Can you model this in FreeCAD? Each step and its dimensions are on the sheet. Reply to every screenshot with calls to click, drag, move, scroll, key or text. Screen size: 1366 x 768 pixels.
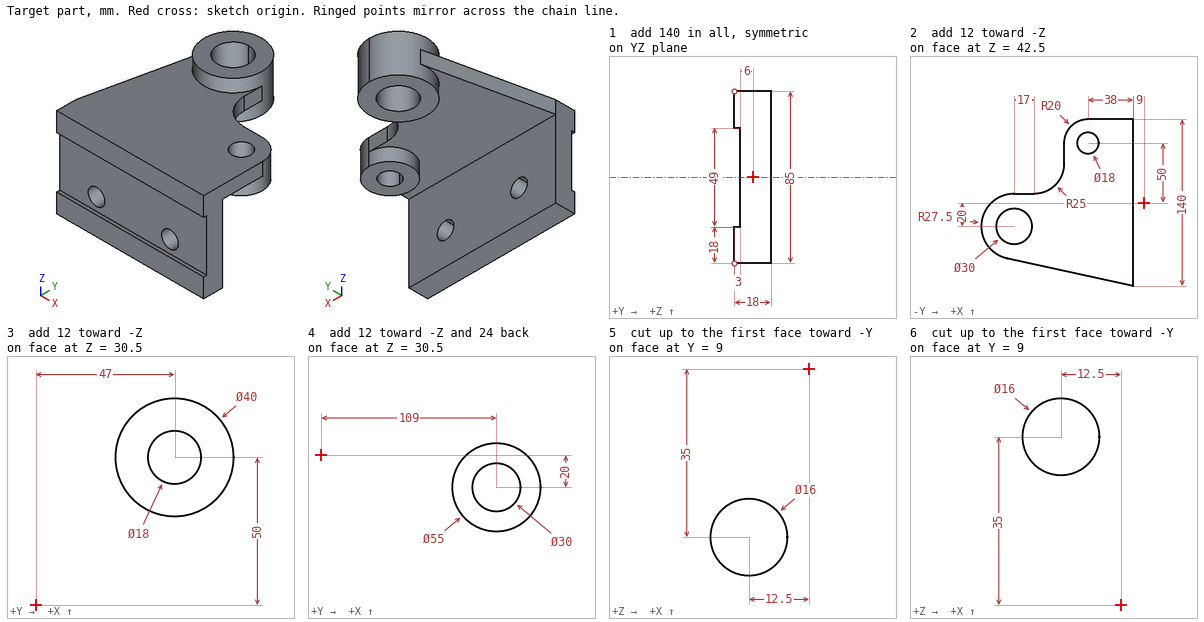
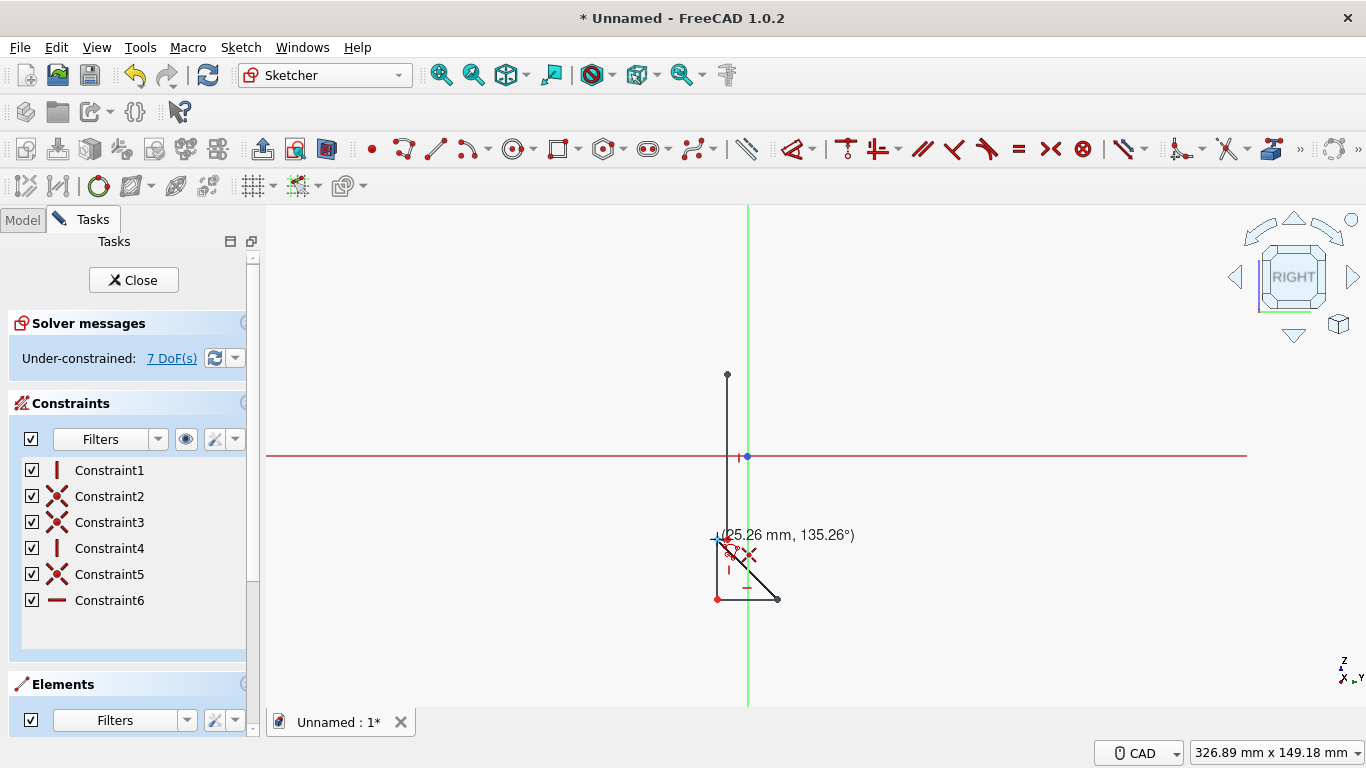
click(778, 313)
click(717, 313)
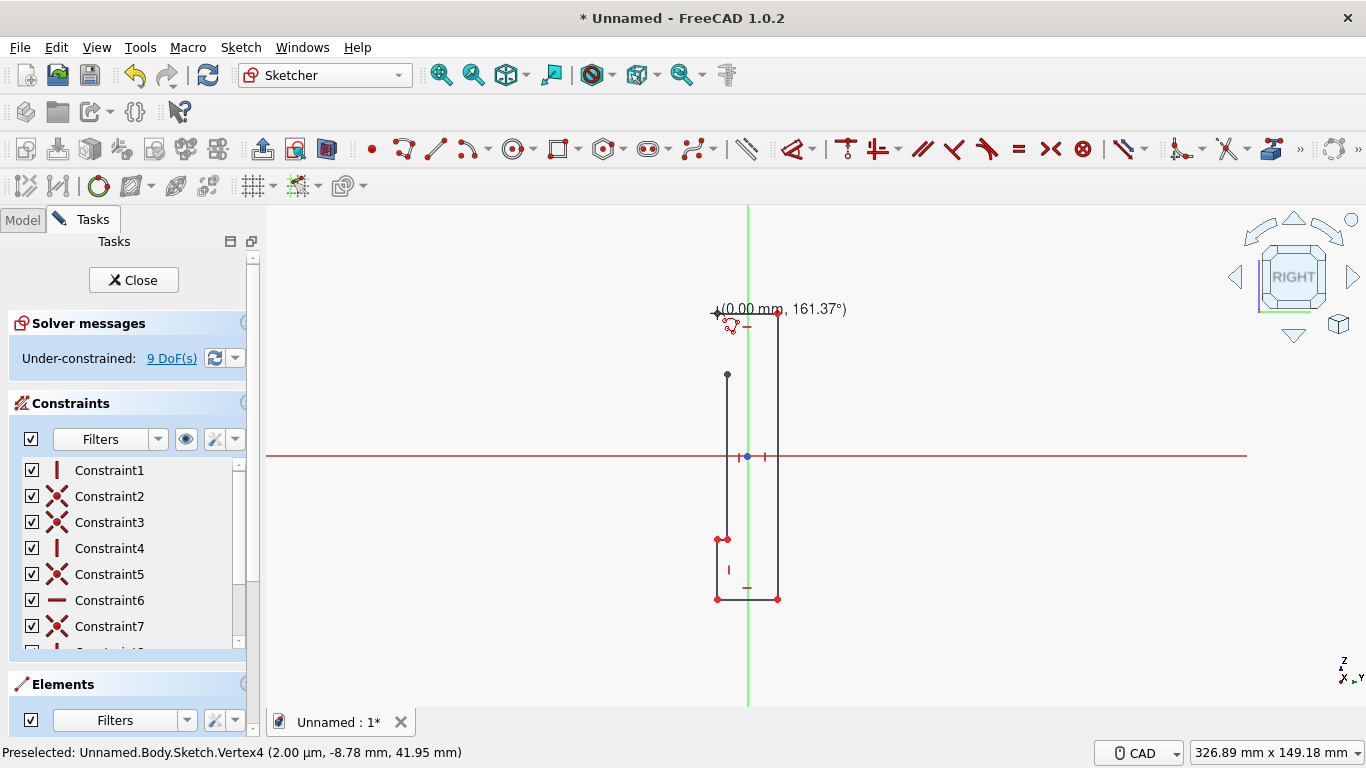
scroll(717, 374, up, 3)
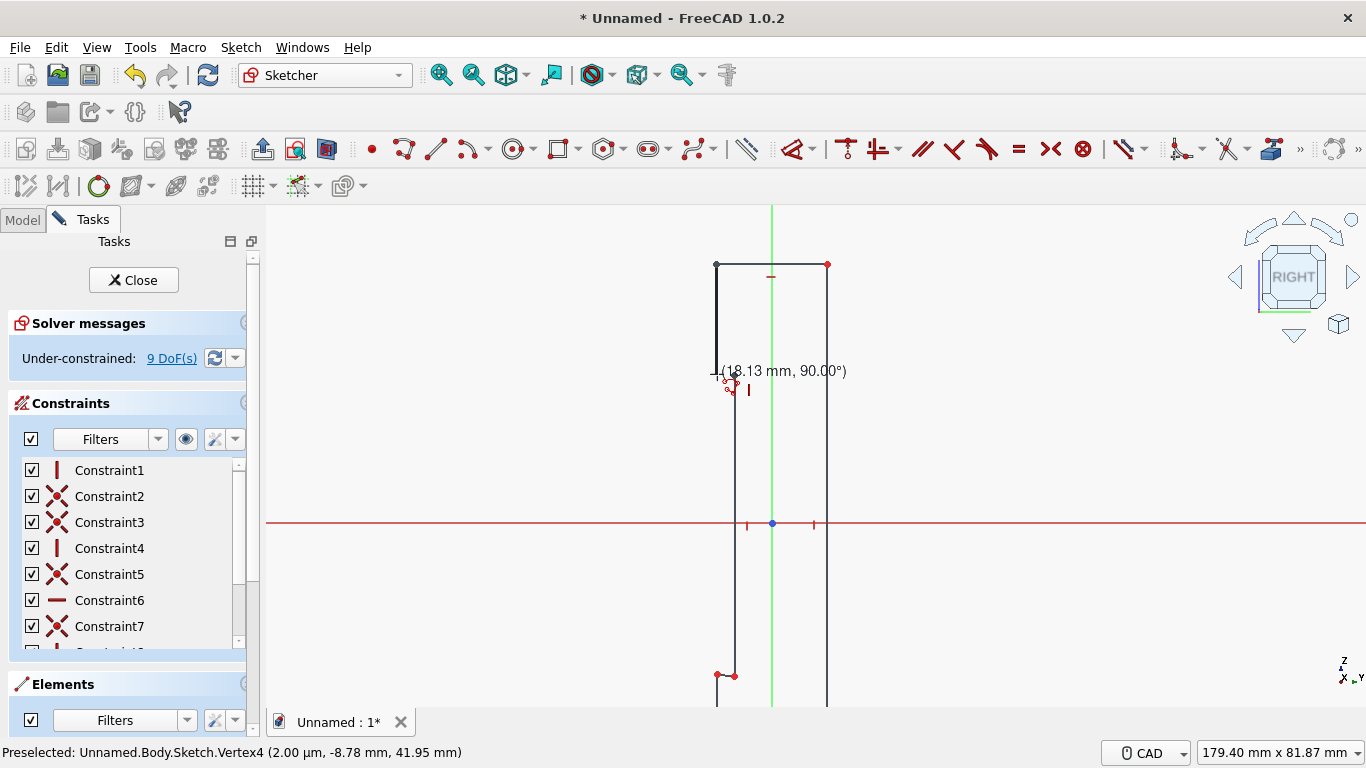
click(717, 373)
click(735, 376)
key(Escape)
key(Escape)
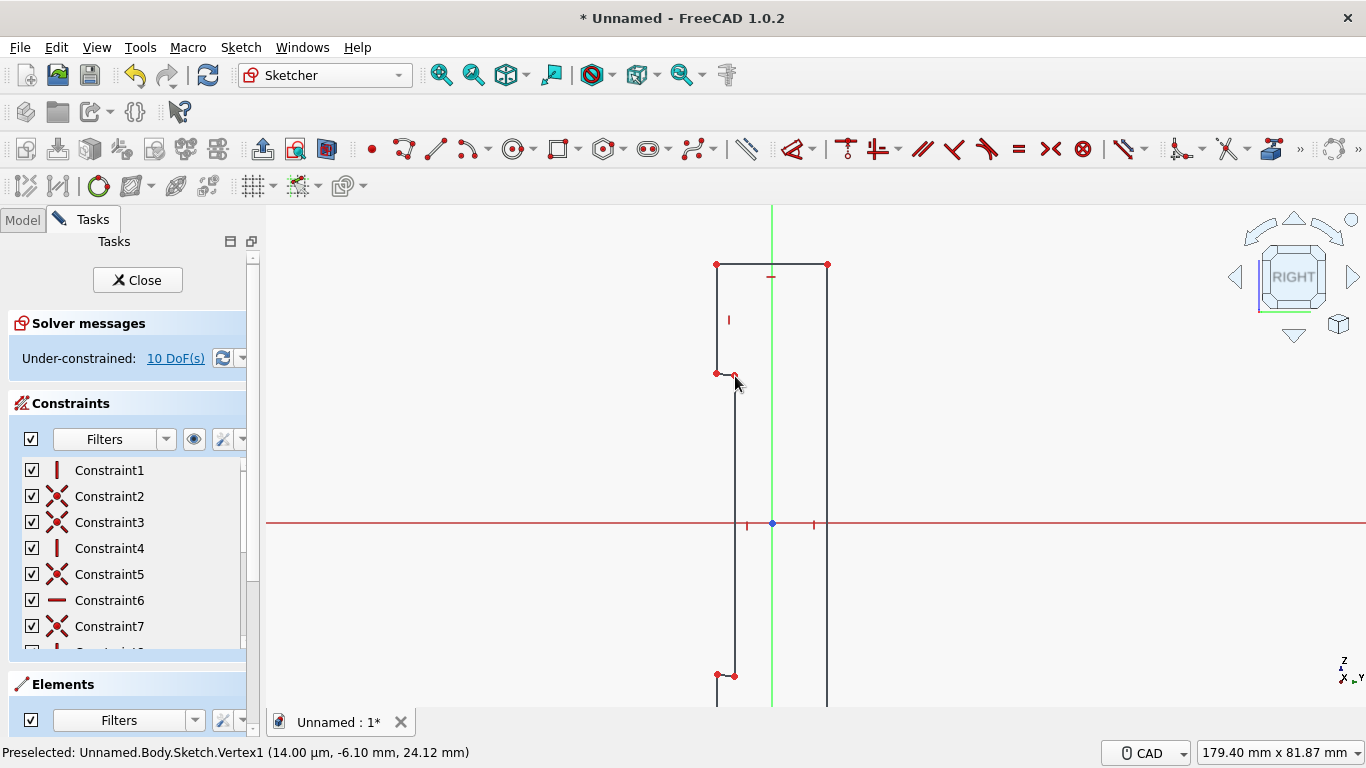
scroll(726, 676, up, 3)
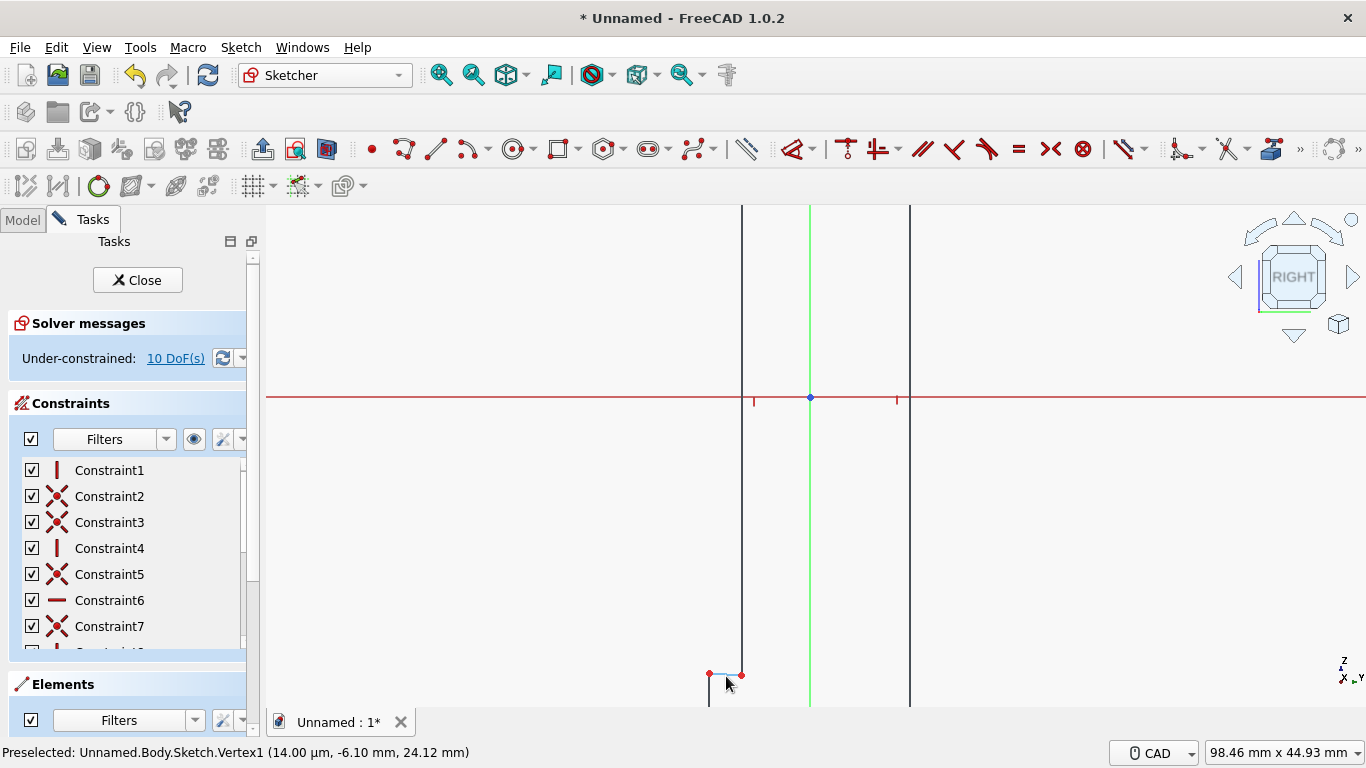
click(726, 674)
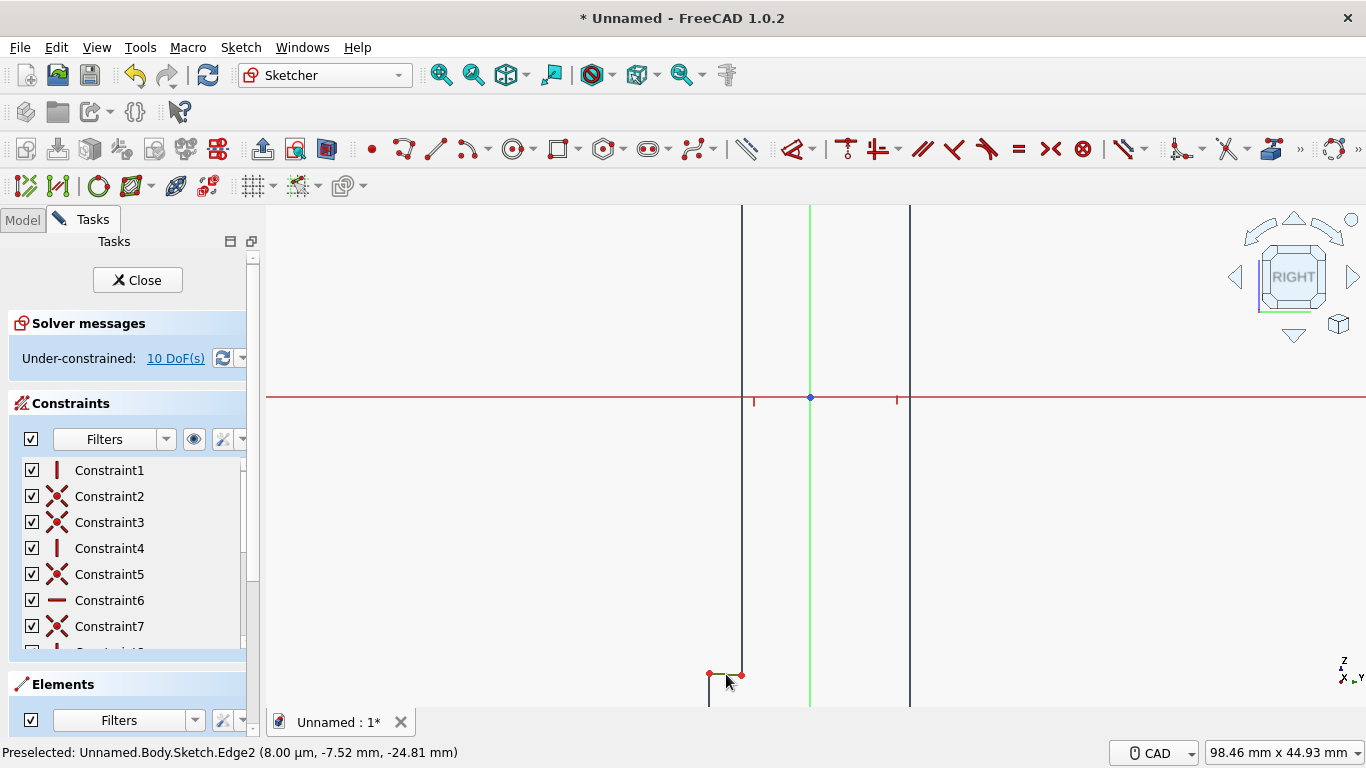
key(h)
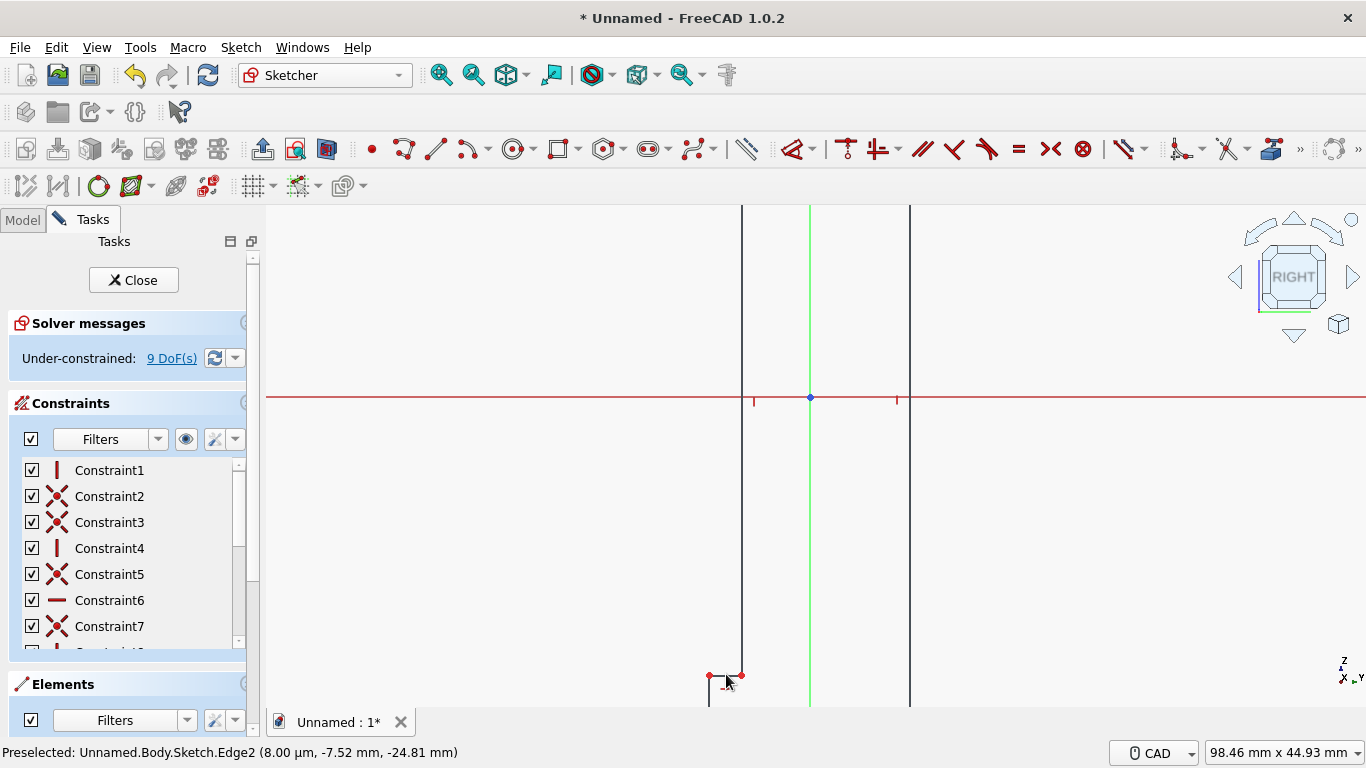
scroll(721, 481, down, 6)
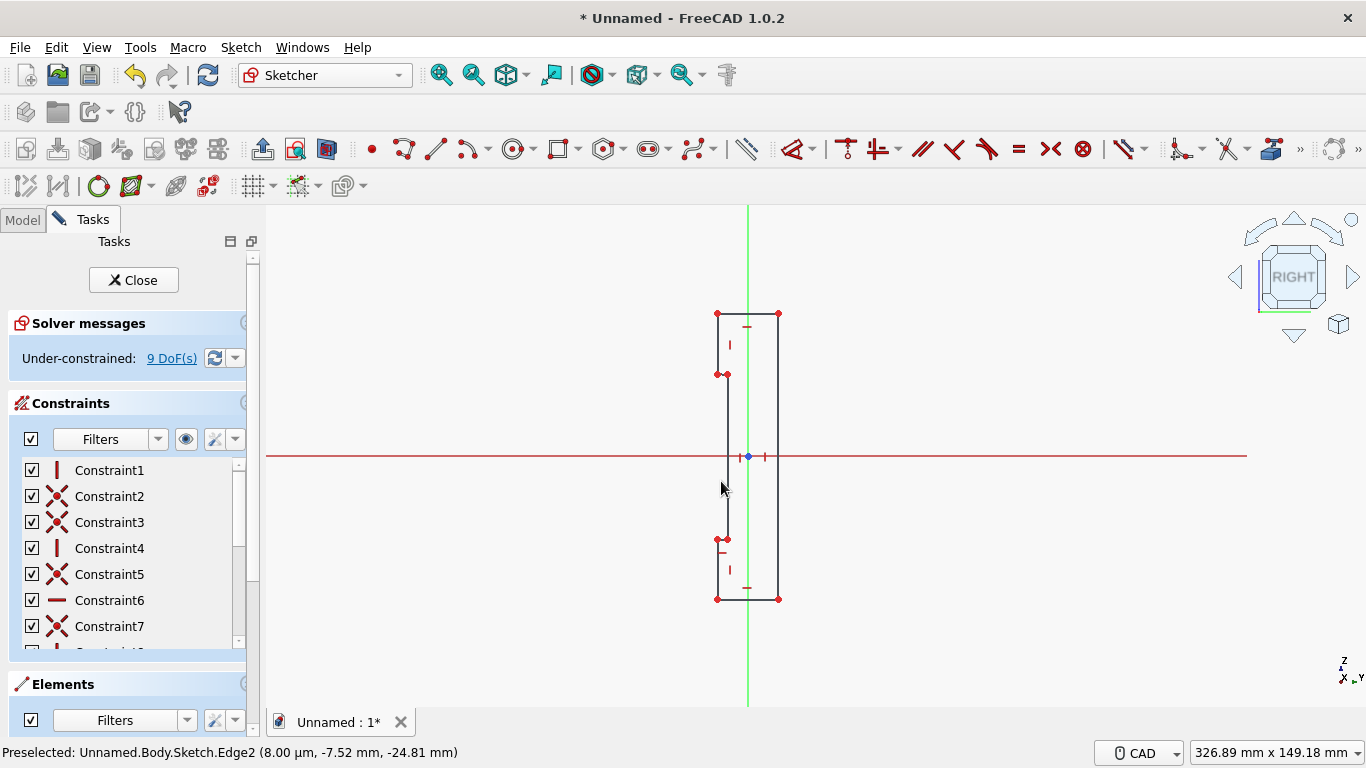
scroll(721, 374, up, 8)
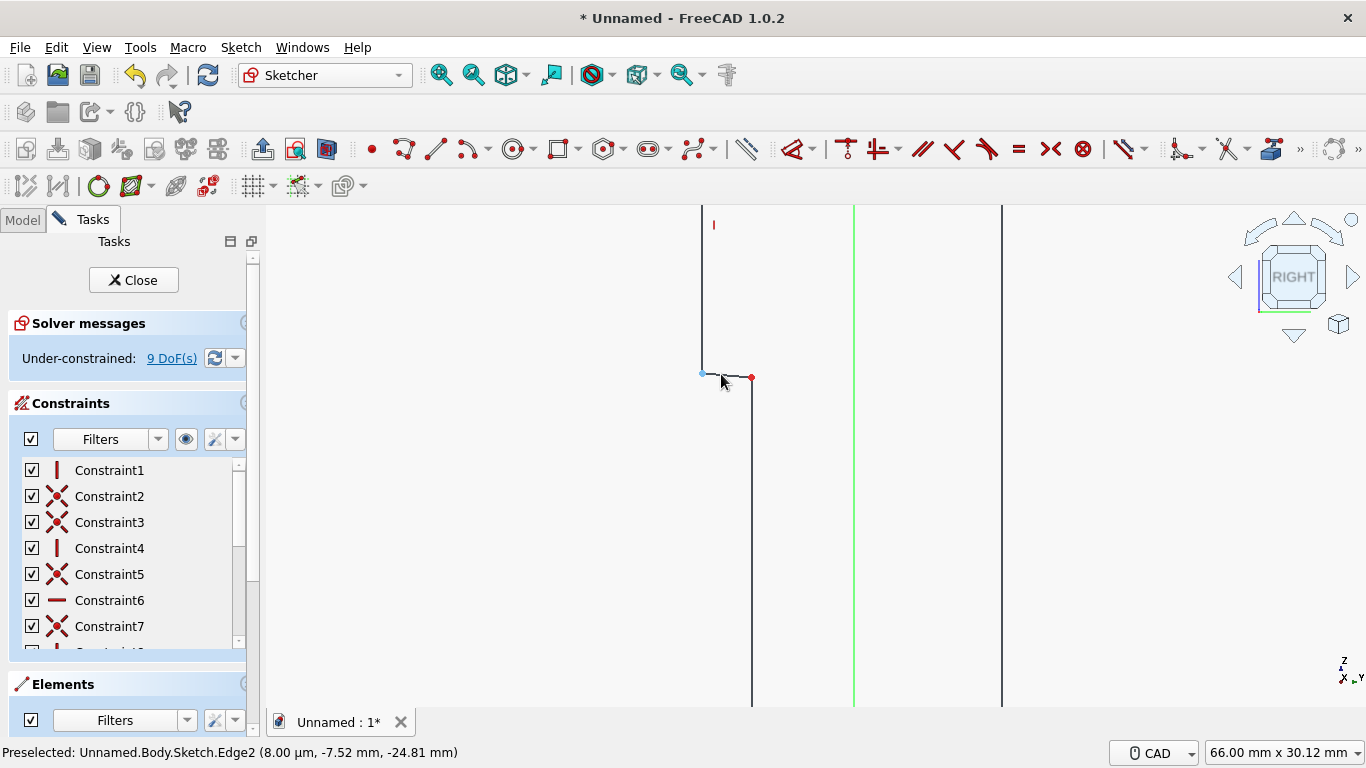
click(717, 375)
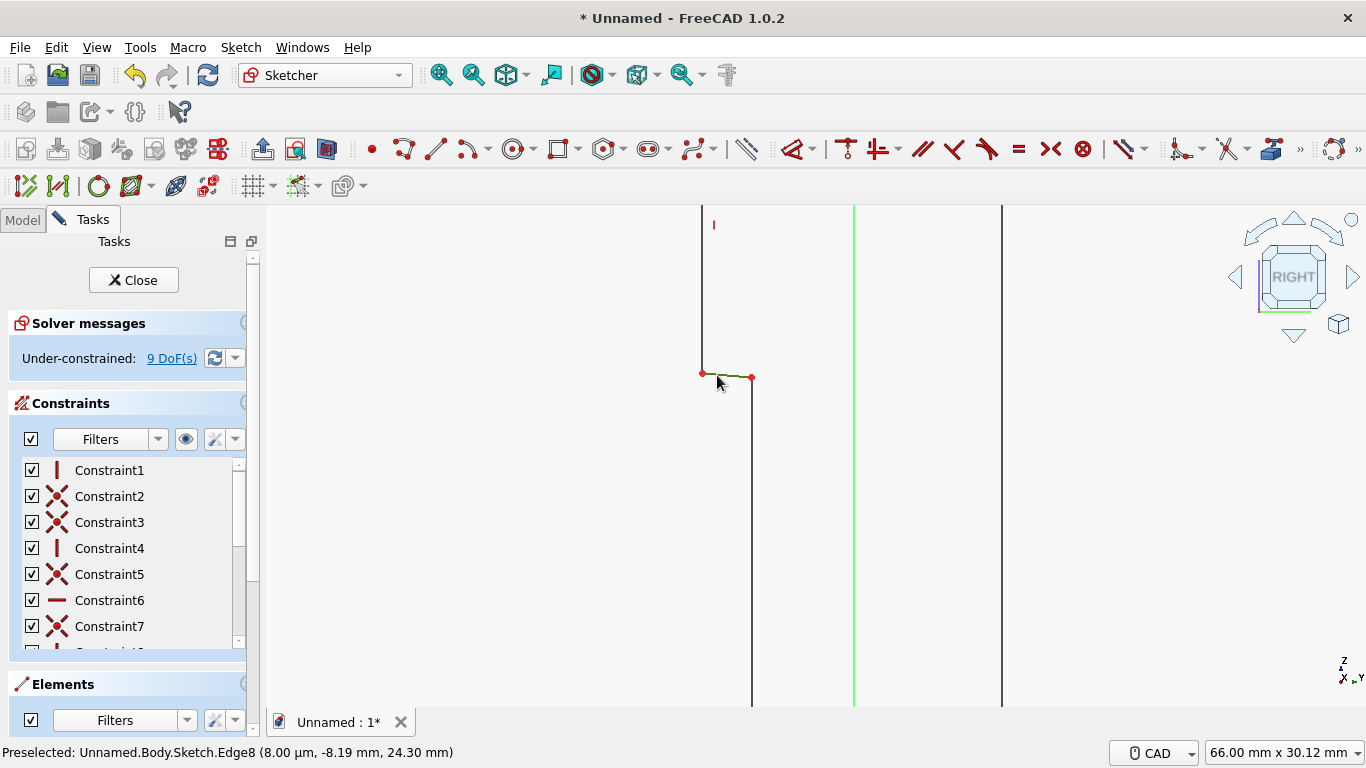
key(h)